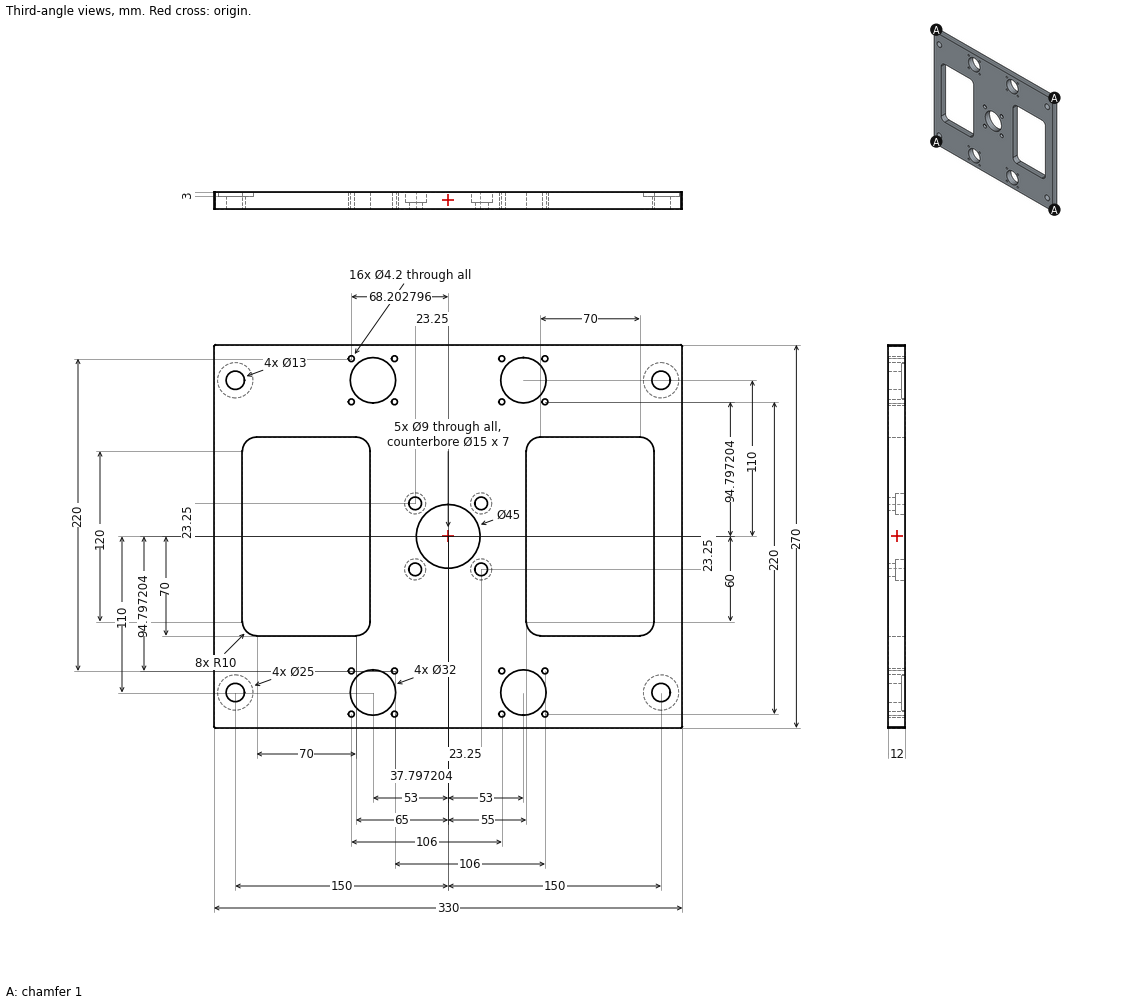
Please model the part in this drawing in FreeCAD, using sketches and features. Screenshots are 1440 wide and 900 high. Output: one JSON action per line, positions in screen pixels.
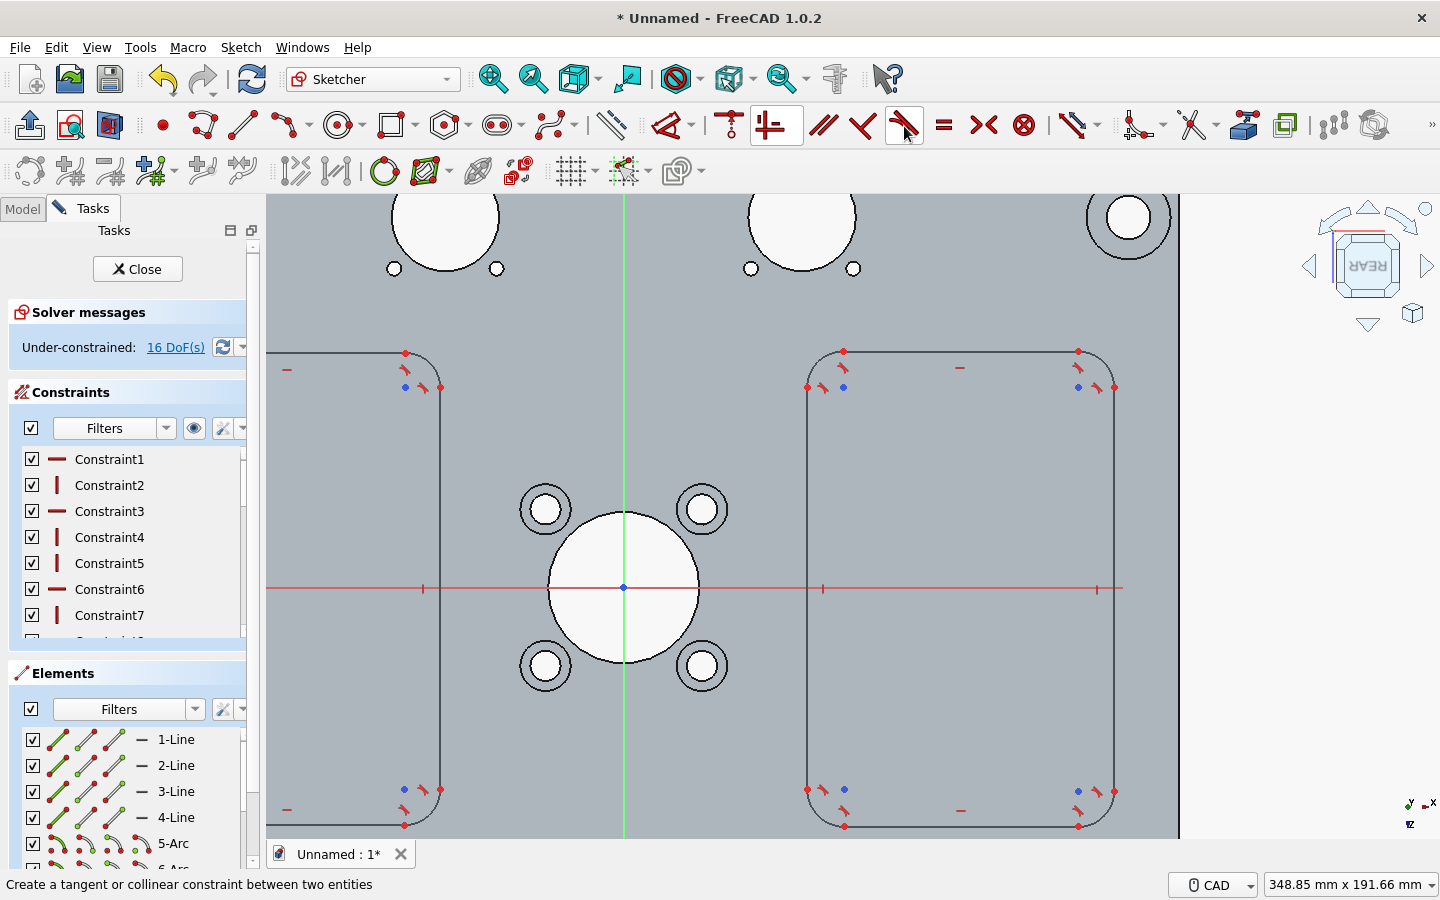
{"action": "scroll", "coordinate": [1111, 372], "scroll_direction": "down", "scroll_amount": 2}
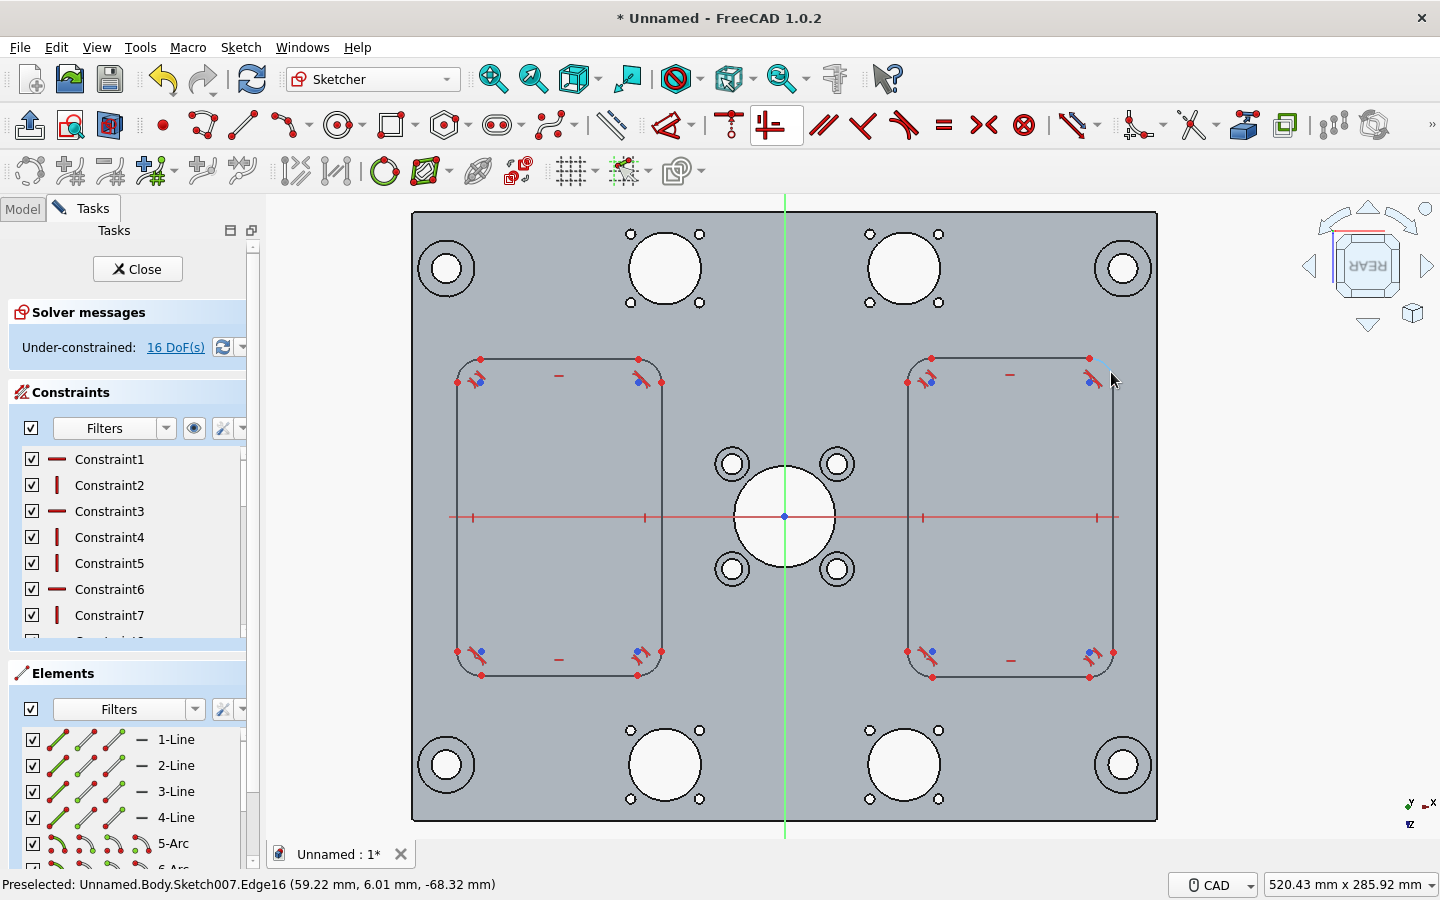
{"action": "scroll", "coordinate": [470, 362], "scroll_direction": "up", "scroll_amount": 2}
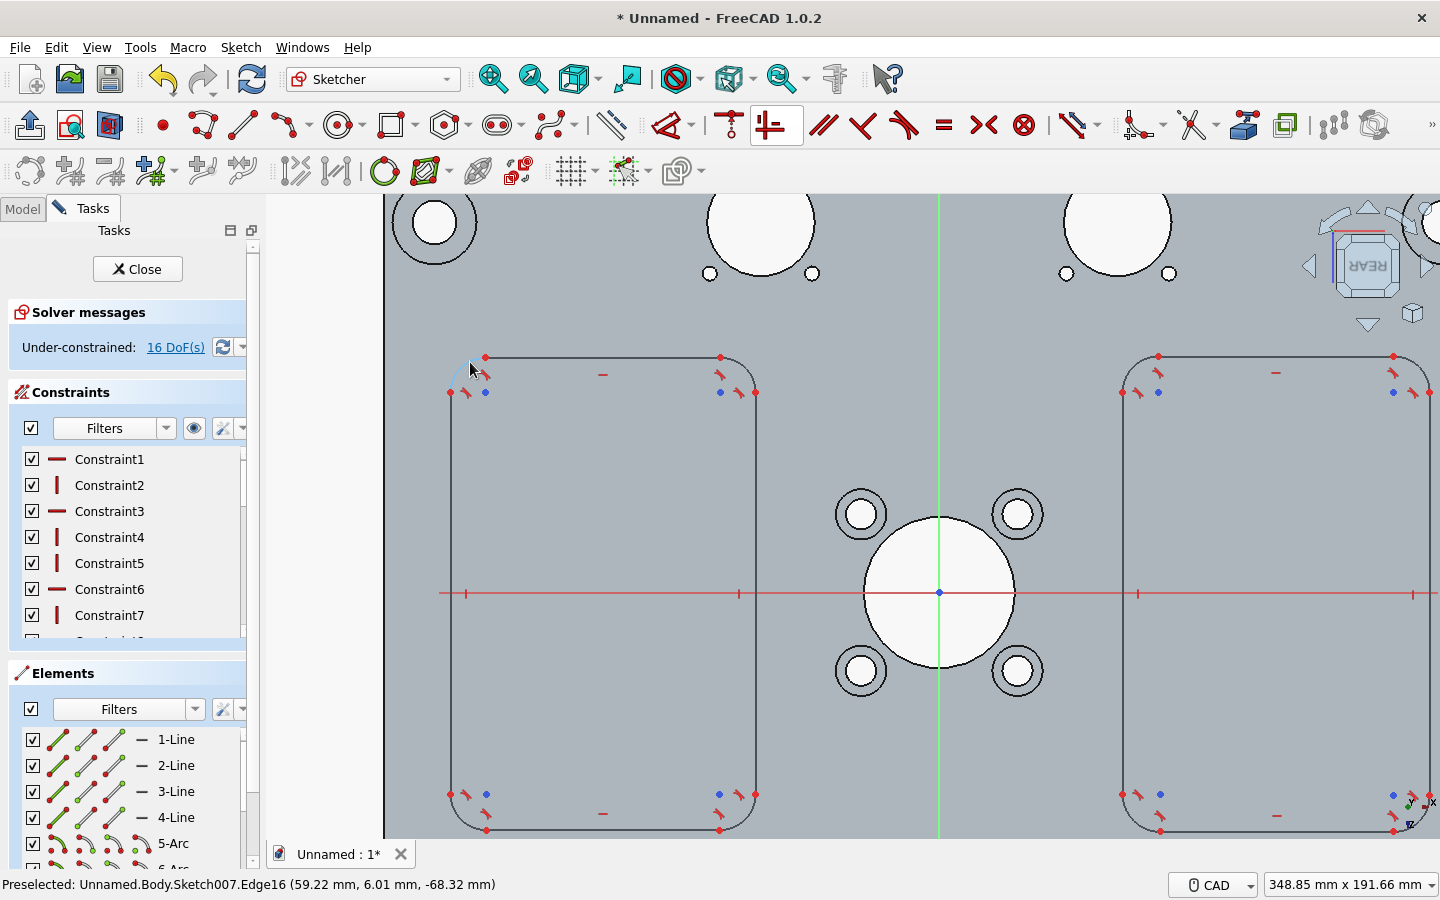
{"action": "left_click", "coordinate": [470, 362]}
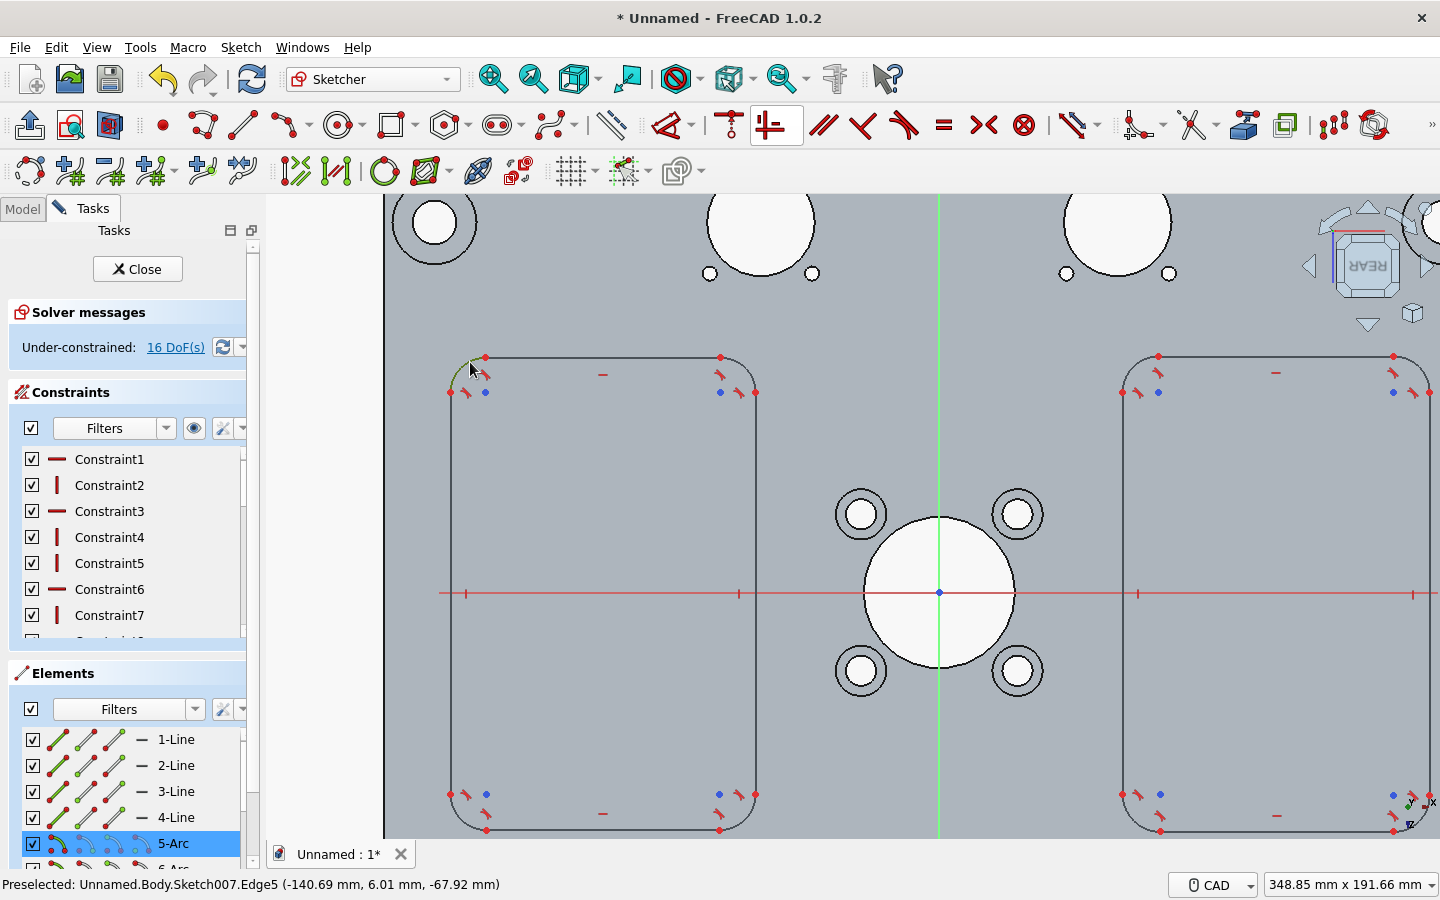
{"action": "left_click", "coordinate": [455, 811]}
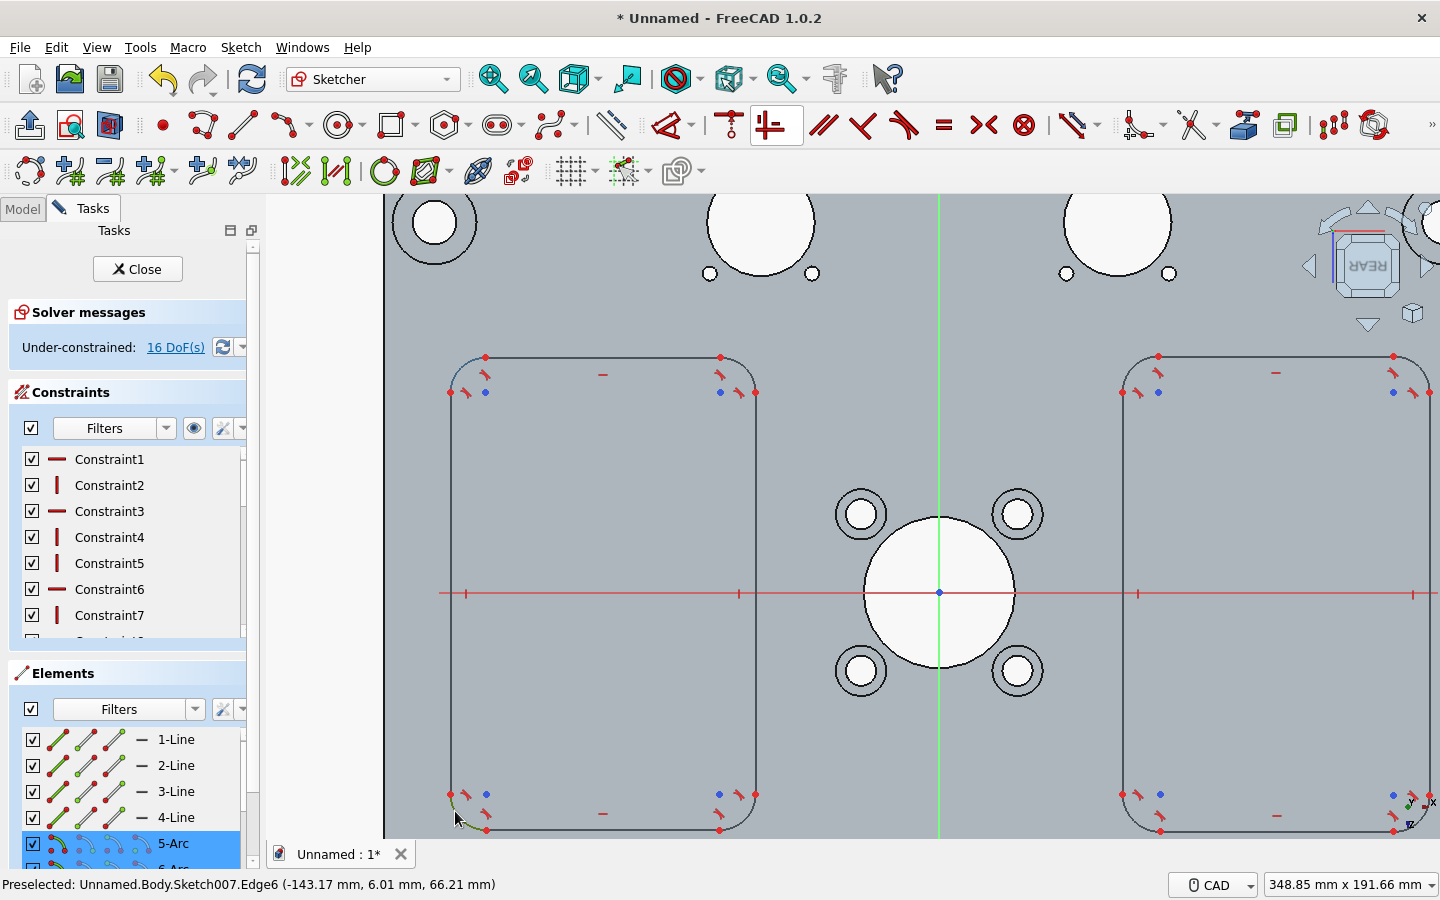
{"action": "left_click", "coordinate": [752, 811]}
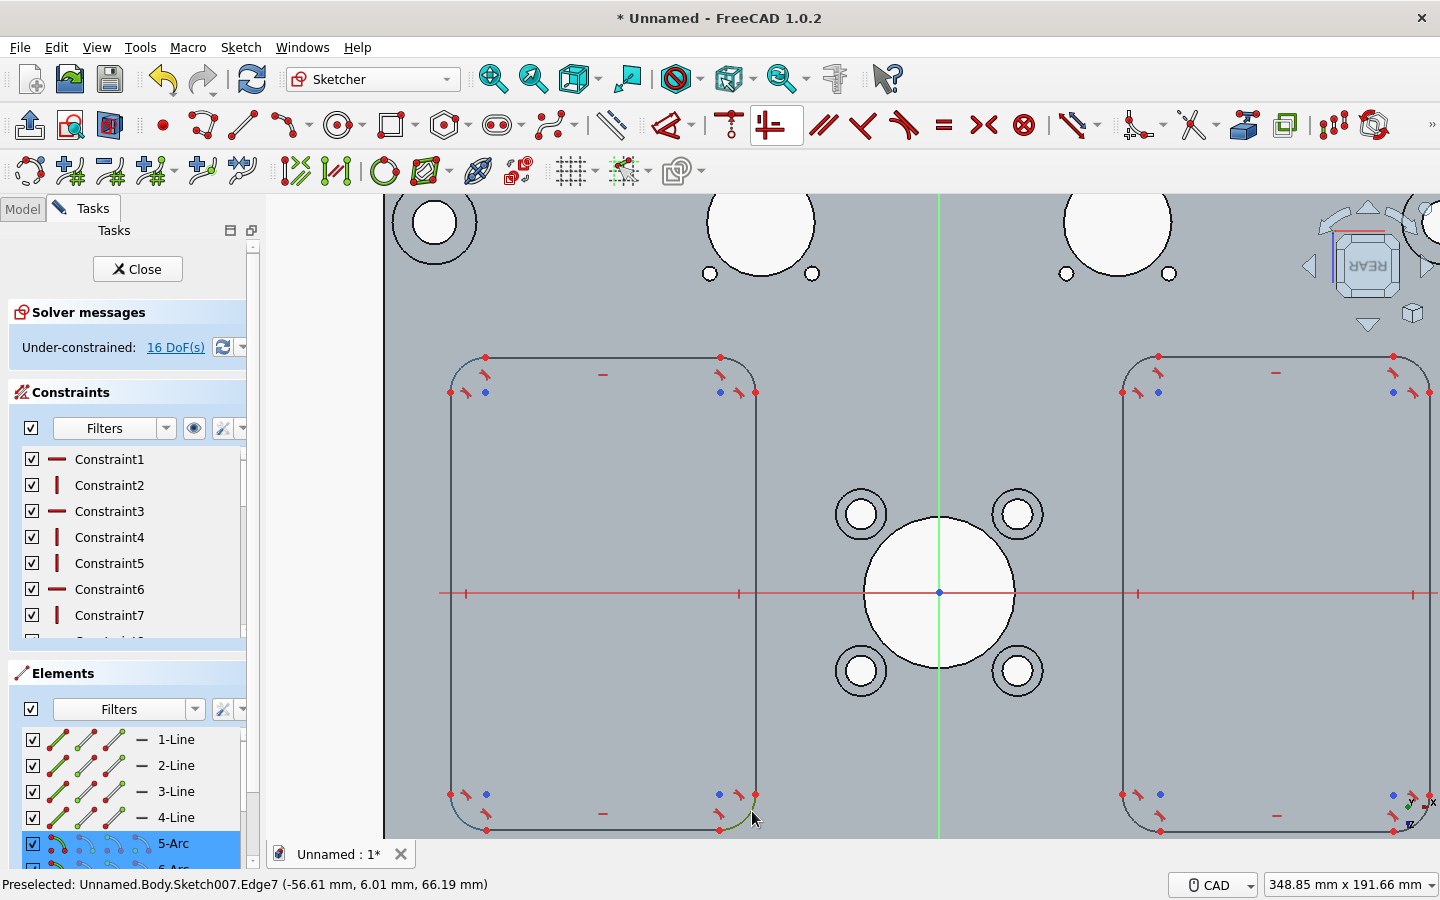
{"action": "left_click", "coordinate": [752, 377]}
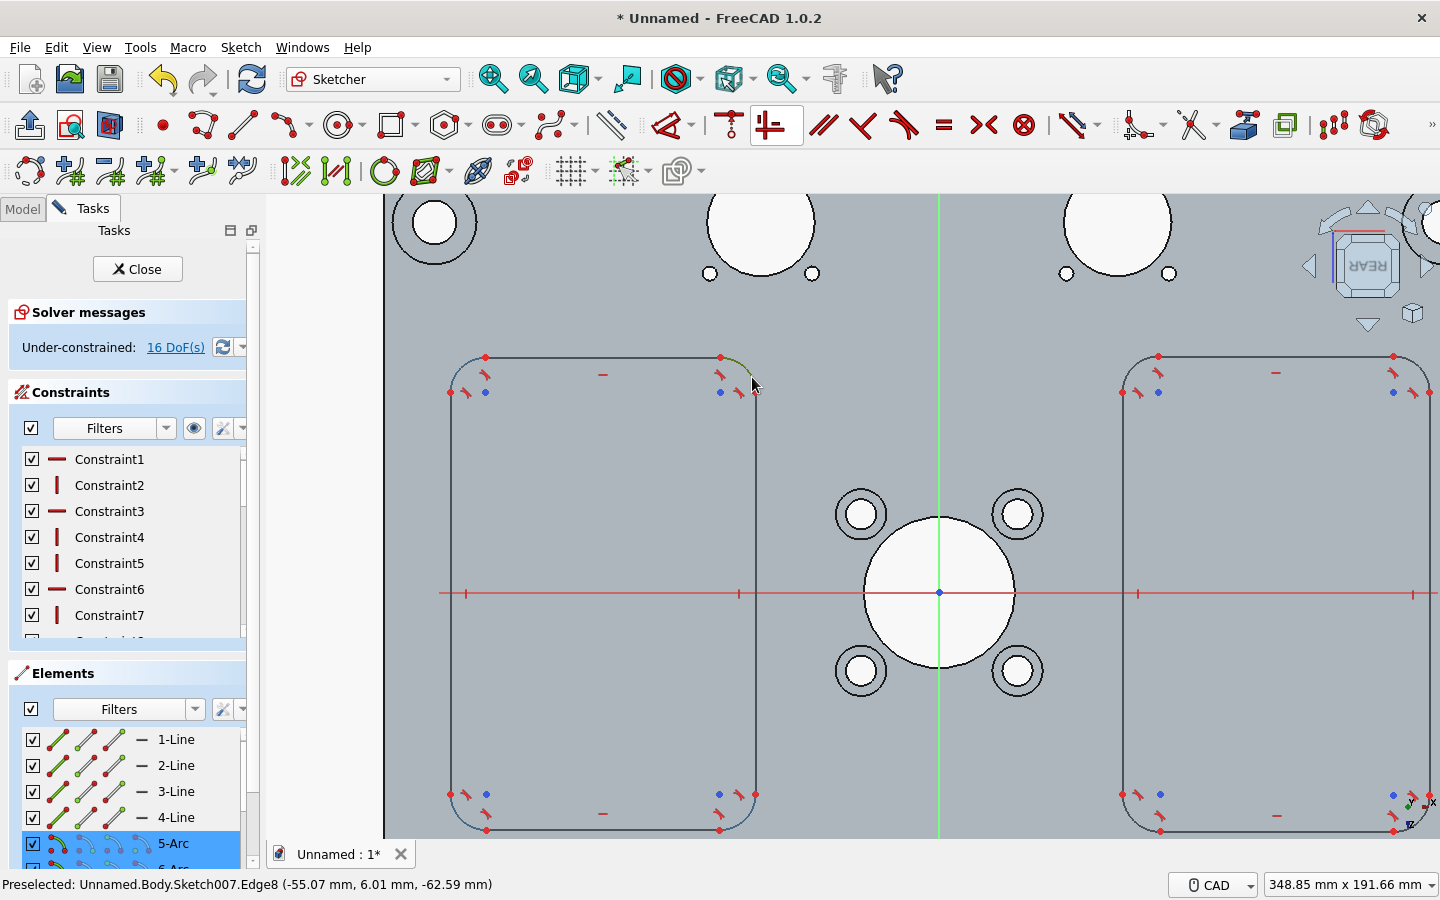
{"action": "left_click", "coordinate": [1125, 806]}